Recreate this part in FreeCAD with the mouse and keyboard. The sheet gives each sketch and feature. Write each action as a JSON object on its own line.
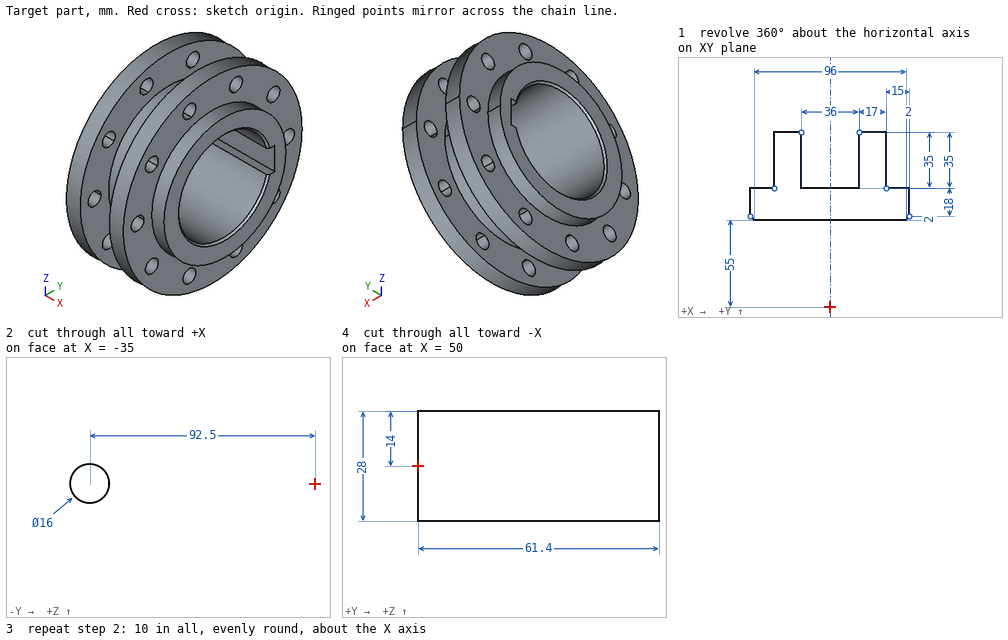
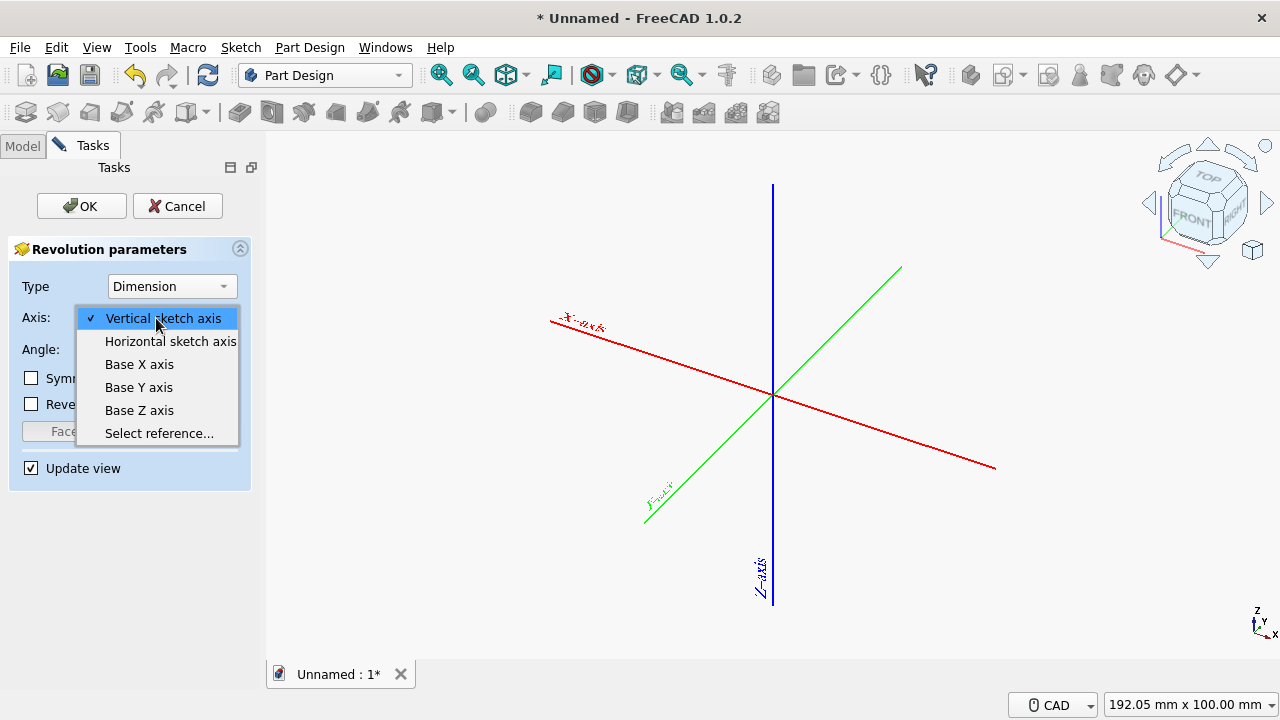
{"action": "left_click", "coordinate": [156, 342]}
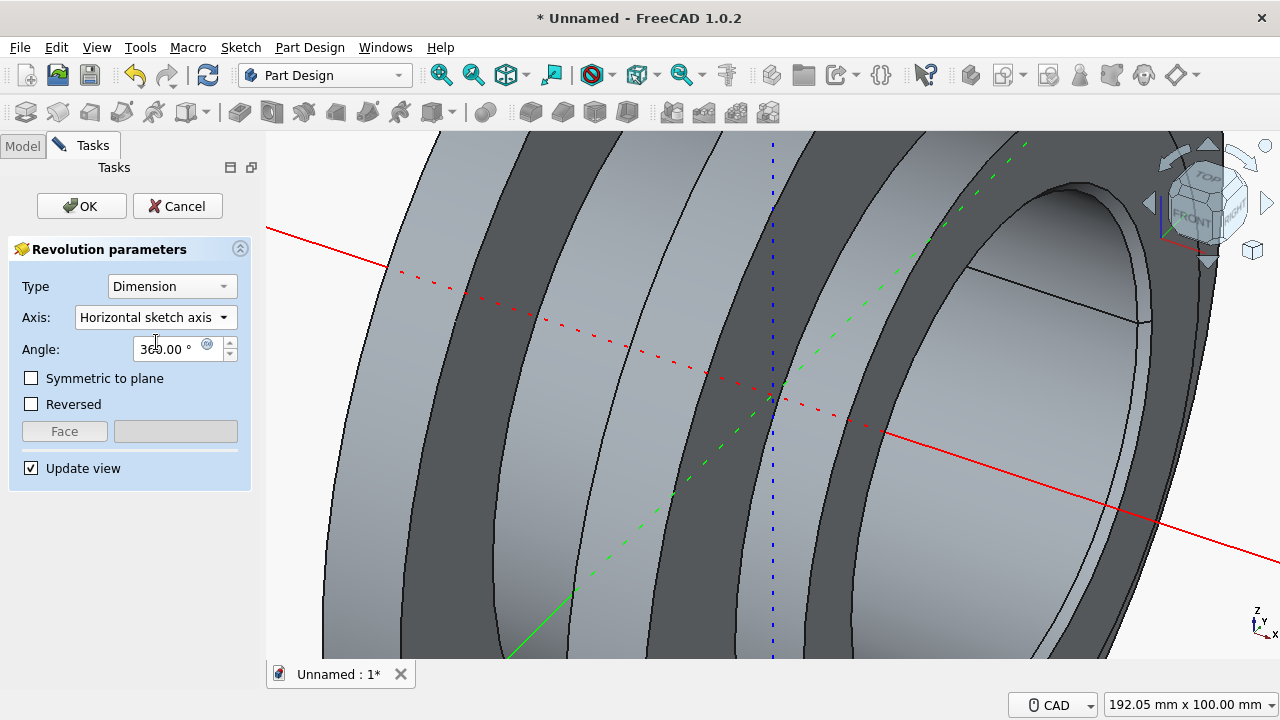
{"action": "left_click", "coordinate": [82, 206]}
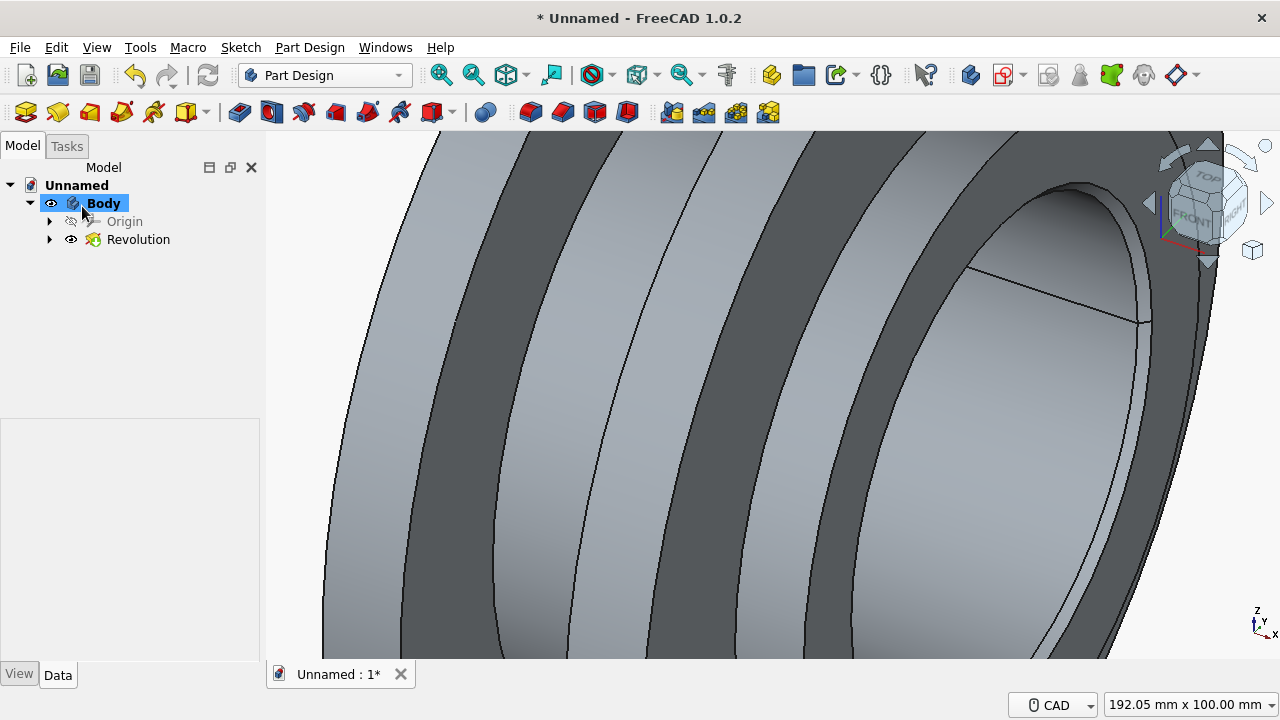
{"action": "left_click", "coordinate": [442, 76]}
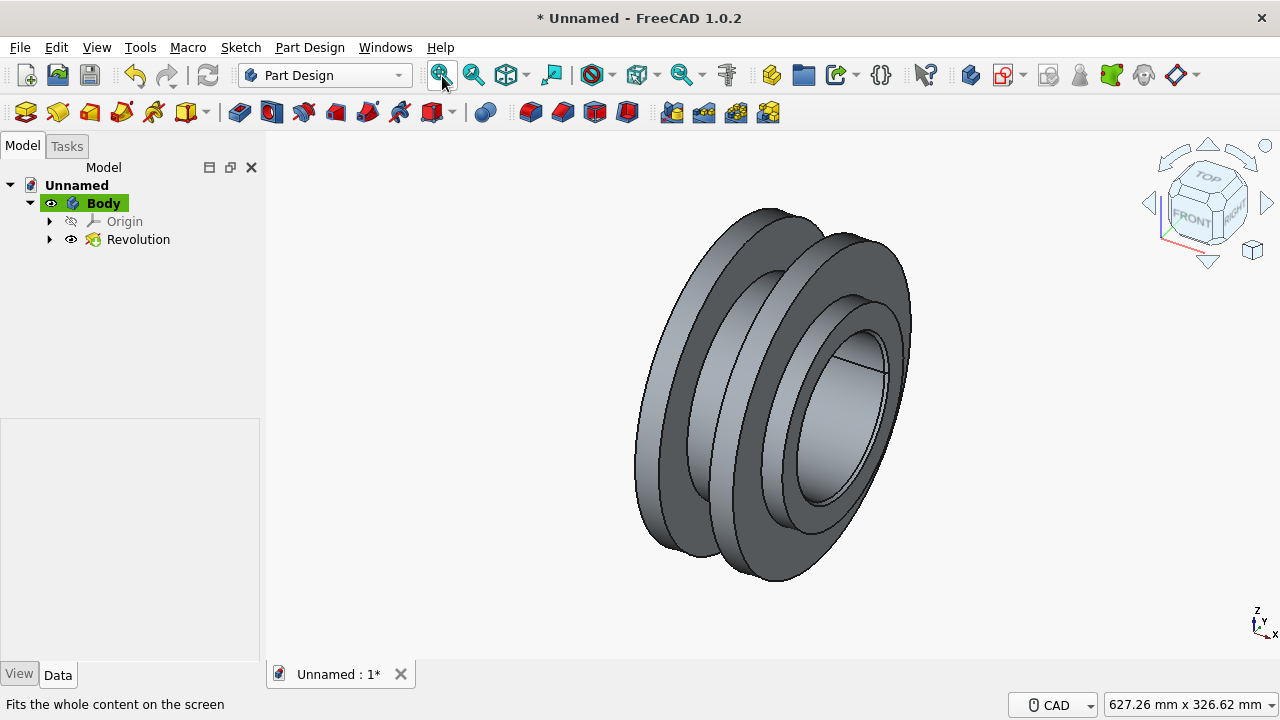
{"action": "key", "text": "6"}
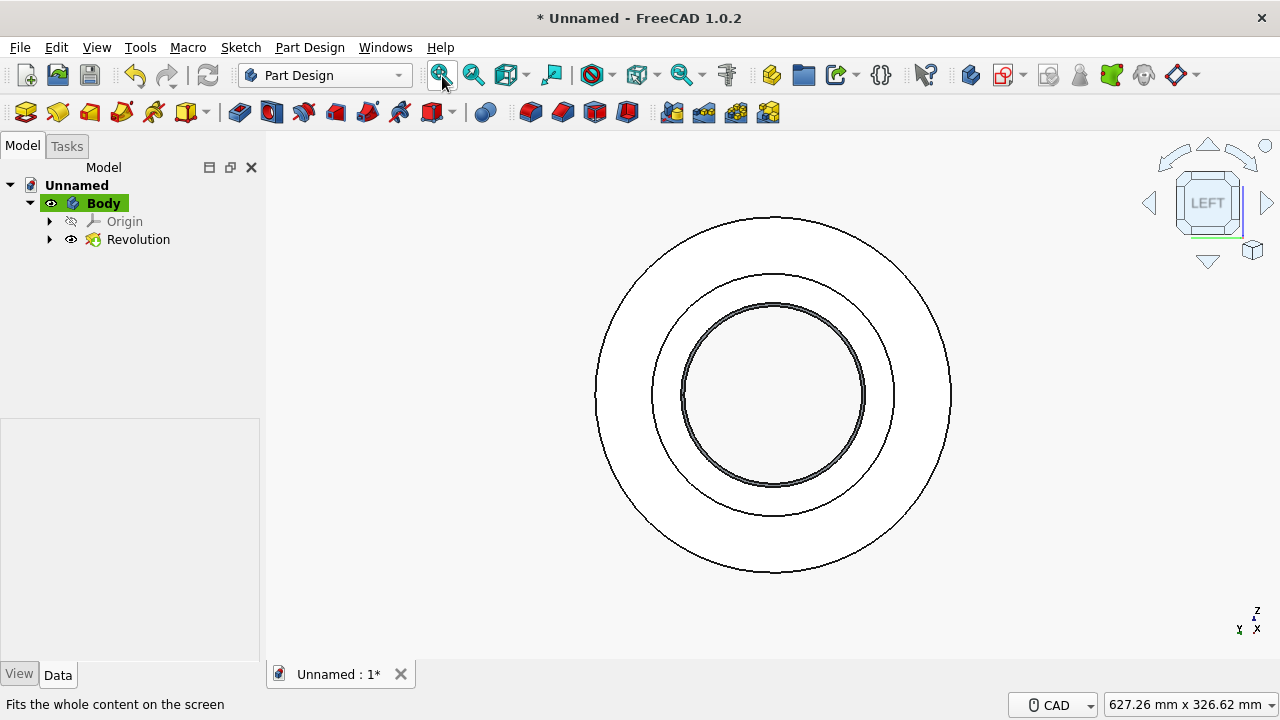
{"action": "left_click", "coordinate": [621, 394]}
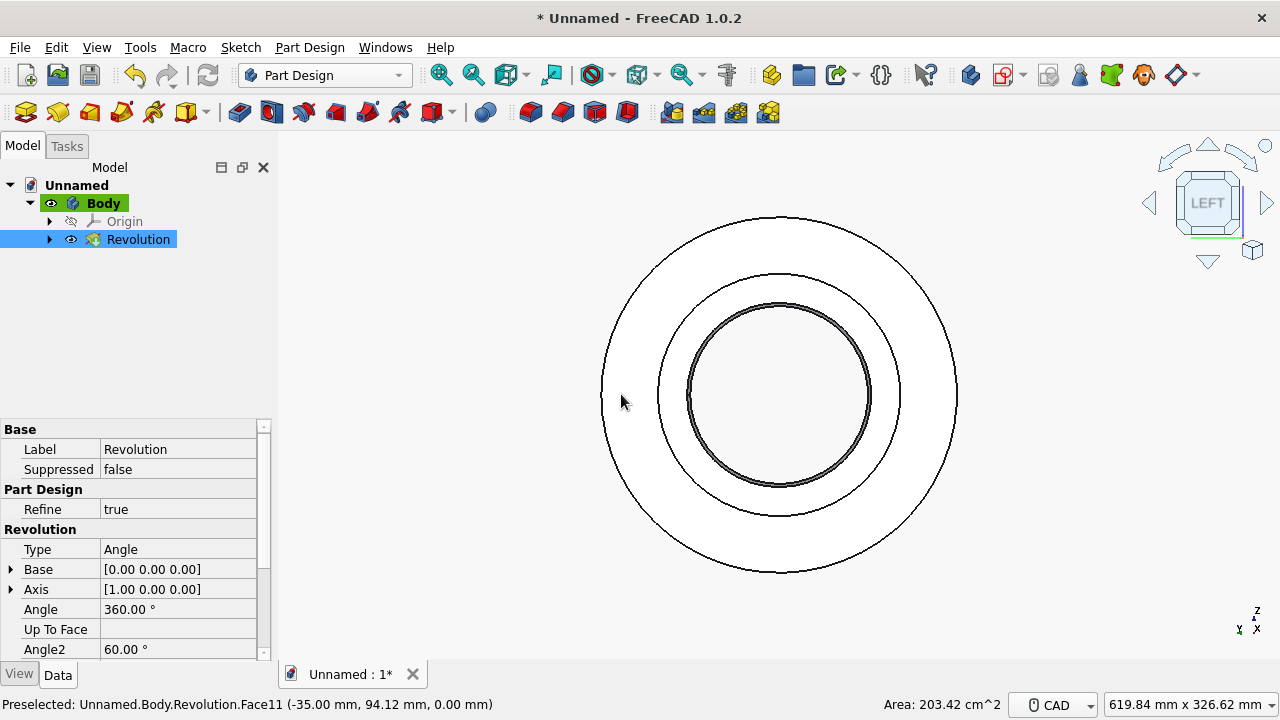
{"action": "left_click", "coordinate": [1004, 76]}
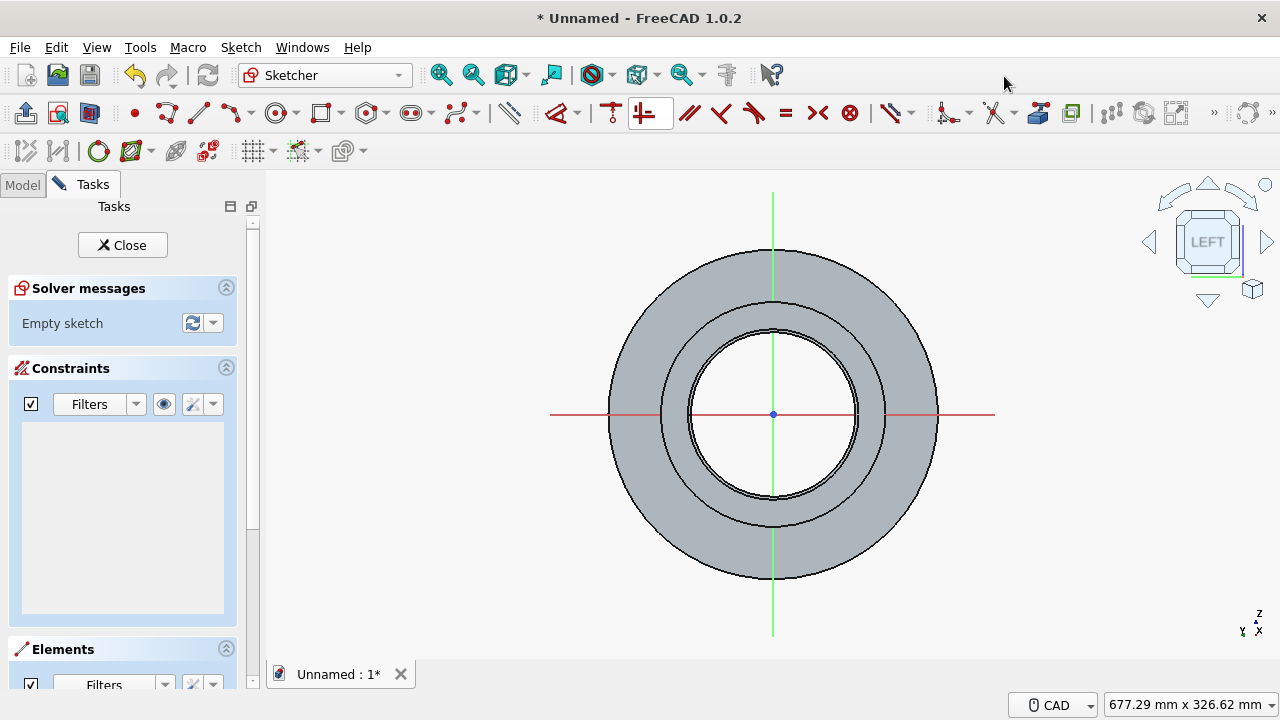
{"action": "scroll", "coordinate": [629, 415], "scroll_direction": "up", "scroll_amount": 13}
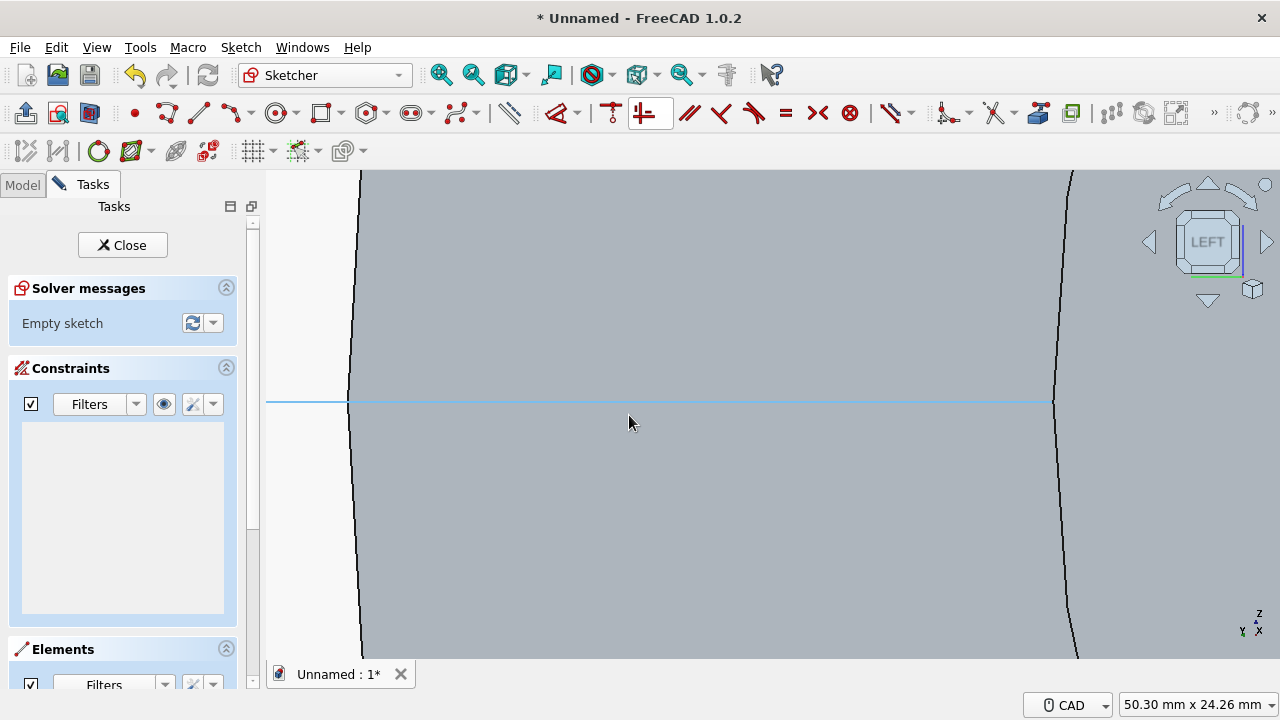
{"action": "left_click", "coordinate": [276, 114]}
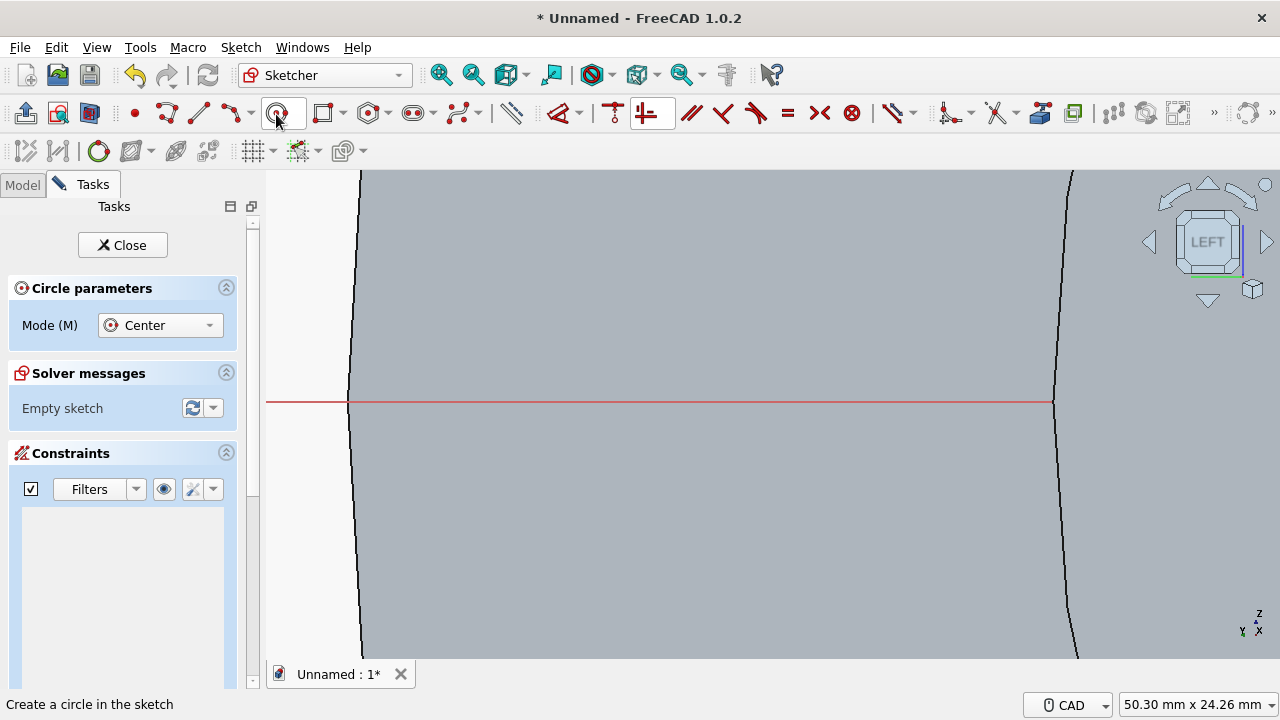
{"action": "left_click", "coordinate": [701, 402]}
{"action": "left_click", "coordinate": [815, 288]}
{"action": "key", "text": "Escape"}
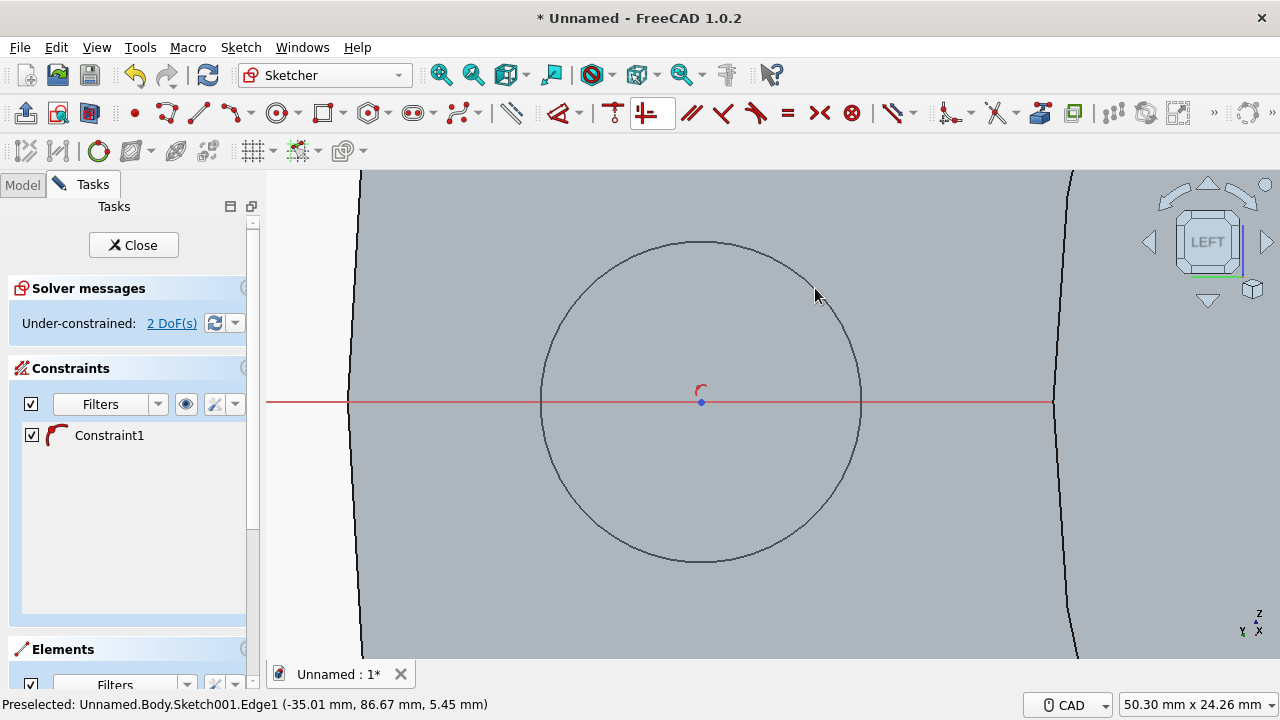
{"action": "left_click", "coordinate": [558, 114]}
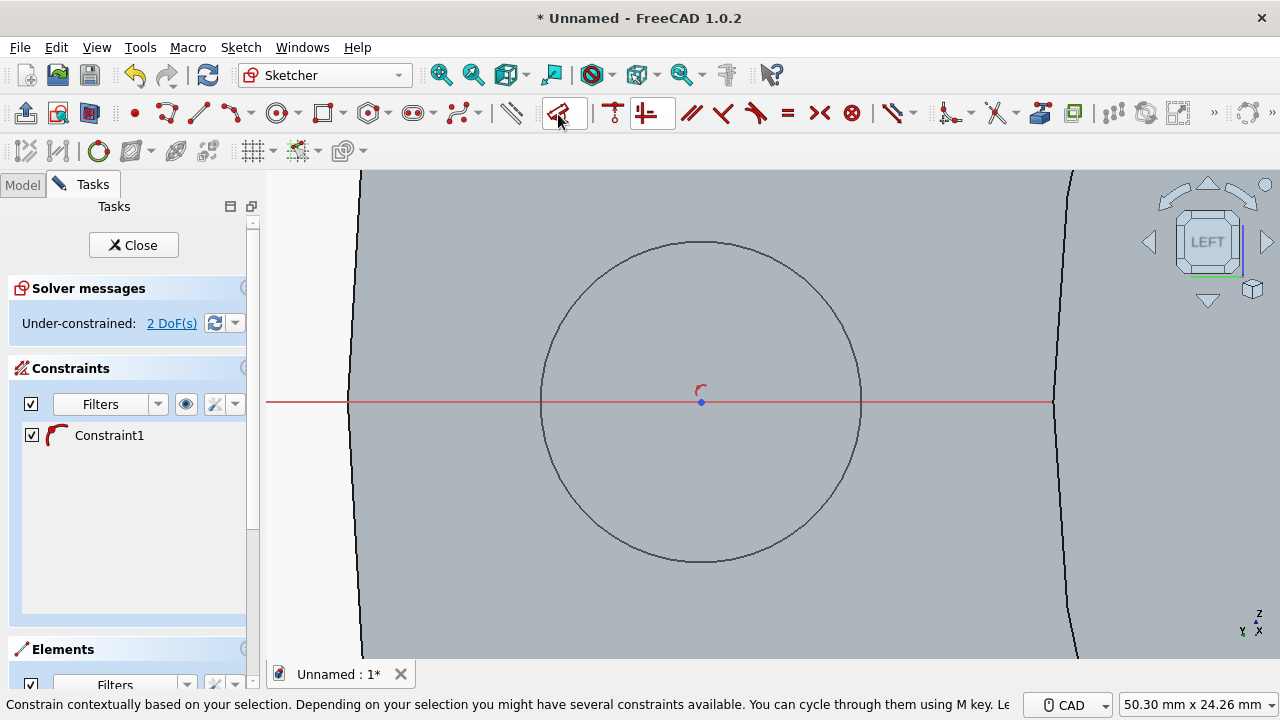
{"action": "left_click", "coordinate": [814, 288]}
{"action": "left_click", "coordinate": [837, 265]}